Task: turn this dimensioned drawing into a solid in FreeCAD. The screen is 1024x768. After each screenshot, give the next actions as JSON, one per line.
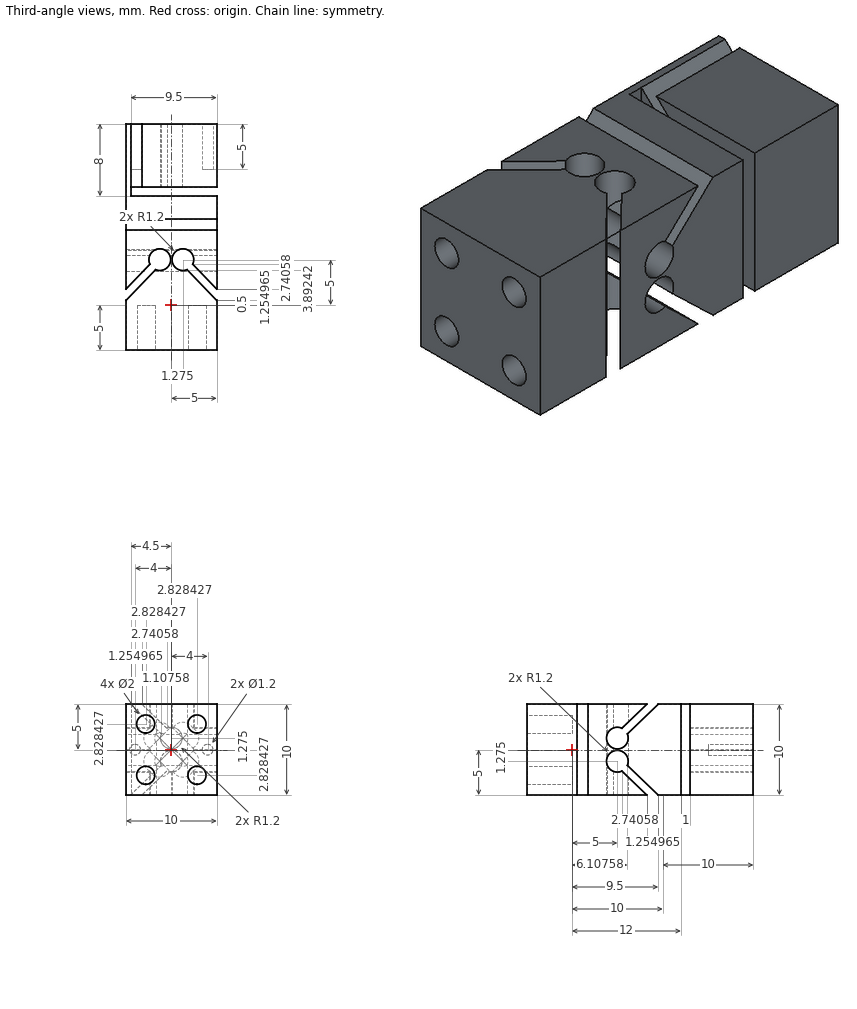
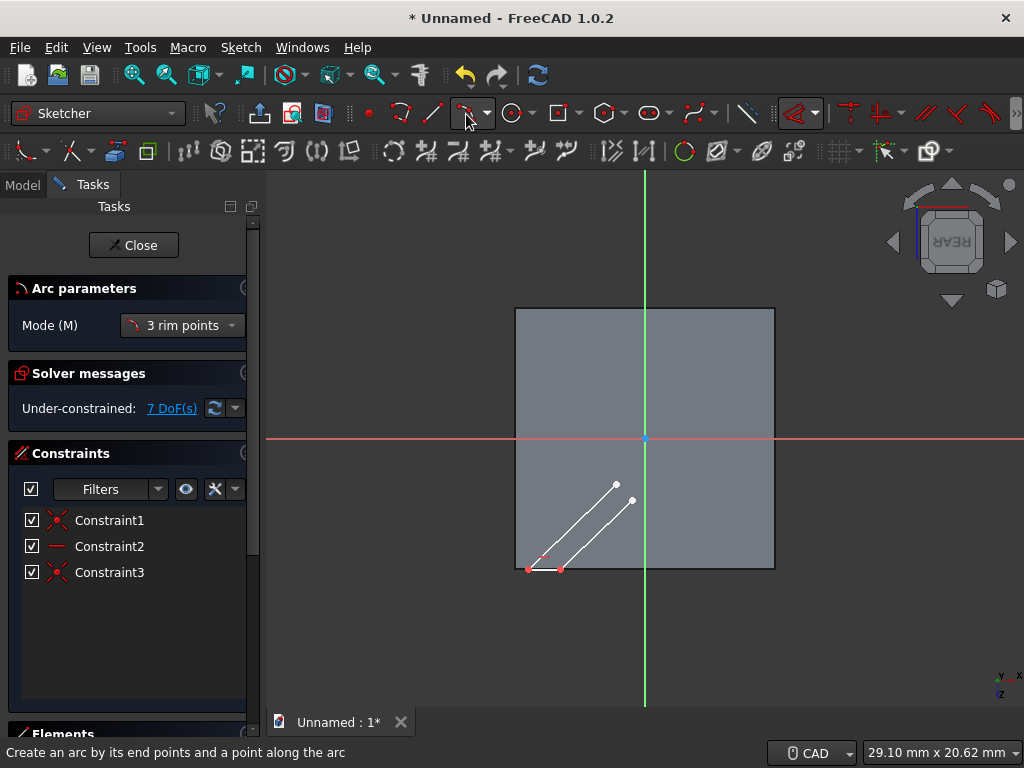
{"action": "left_click", "coordinate": [632, 501]}
{"action": "left_click", "coordinate": [616, 485]}
{"action": "left_click", "coordinate": [676, 465]}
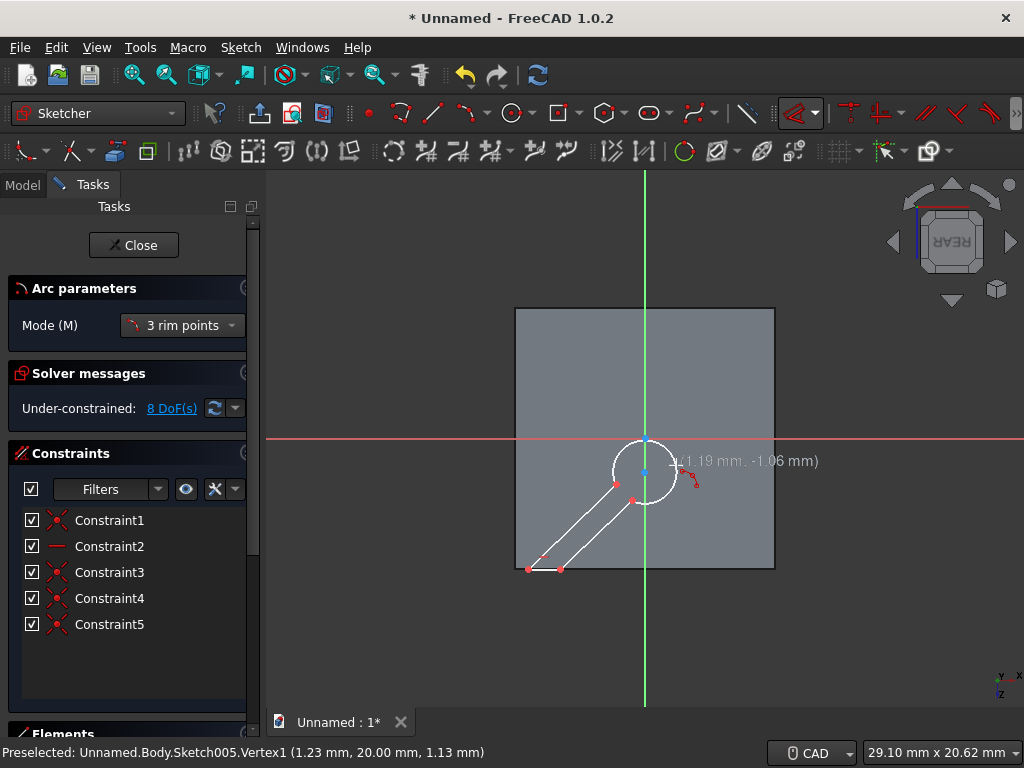
{"action": "left_click", "coordinate": [402, 114]}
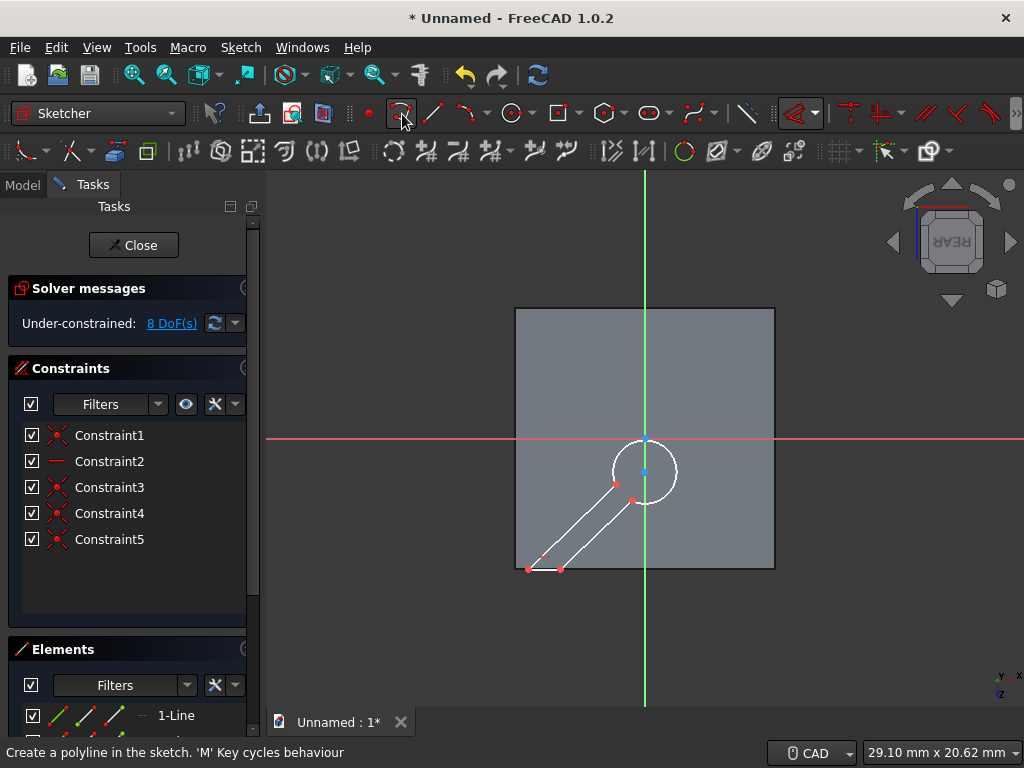
{"action": "left_click", "coordinate": [632, 377]}
{"action": "left_click", "coordinate": [560, 308]}
{"action": "left_click", "coordinate": [528, 308]}
{"action": "left_click", "coordinate": [616, 393]}
{"action": "right_click", "coordinate": [616, 393]}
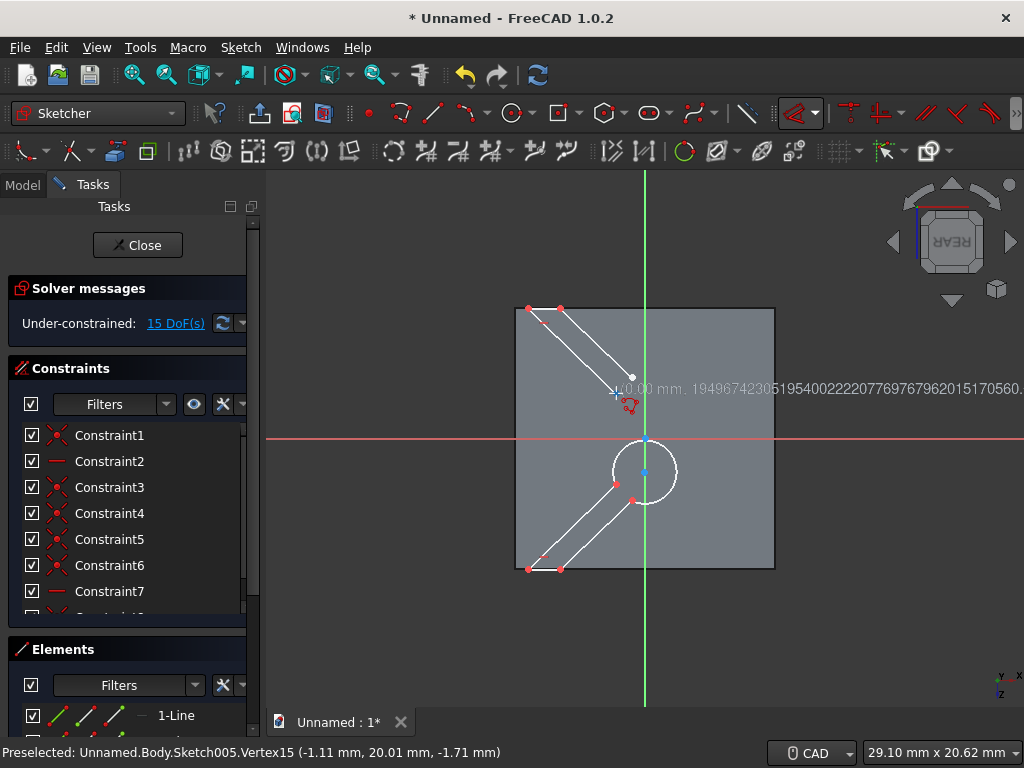
{"action": "left_click", "coordinate": [466, 114]}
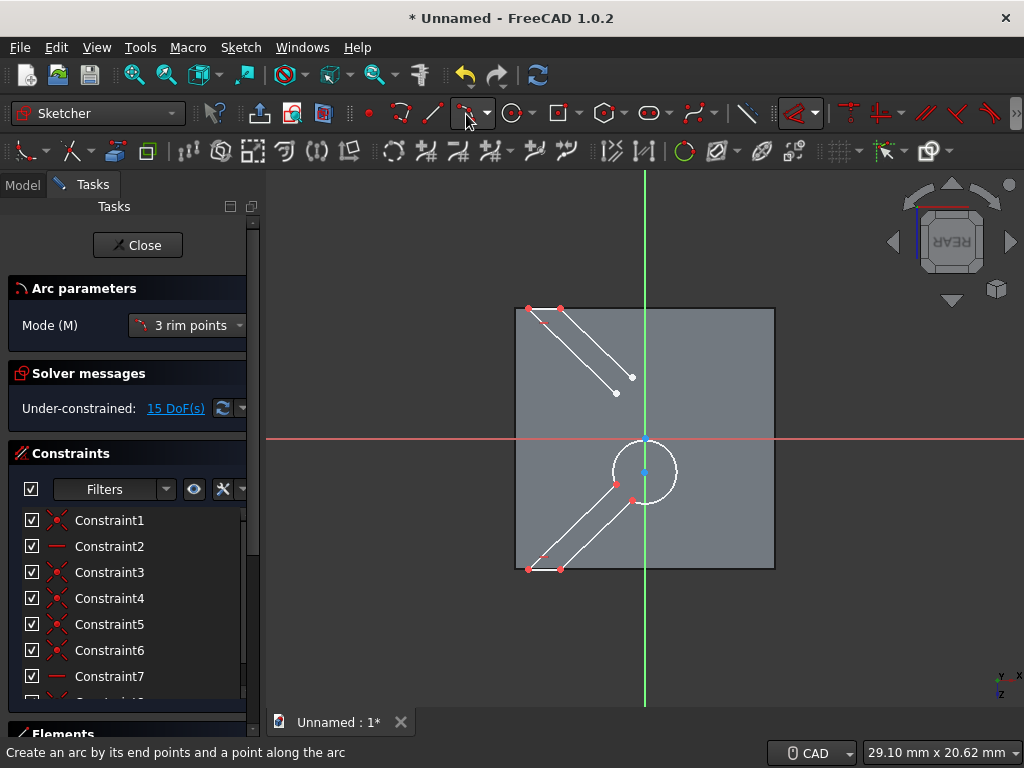
{"action": "left_click", "coordinate": [616, 394]}
{"action": "left_click", "coordinate": [632, 378]}
{"action": "left_click", "coordinate": [676, 412]}
{"action": "key", "text": "Escape"}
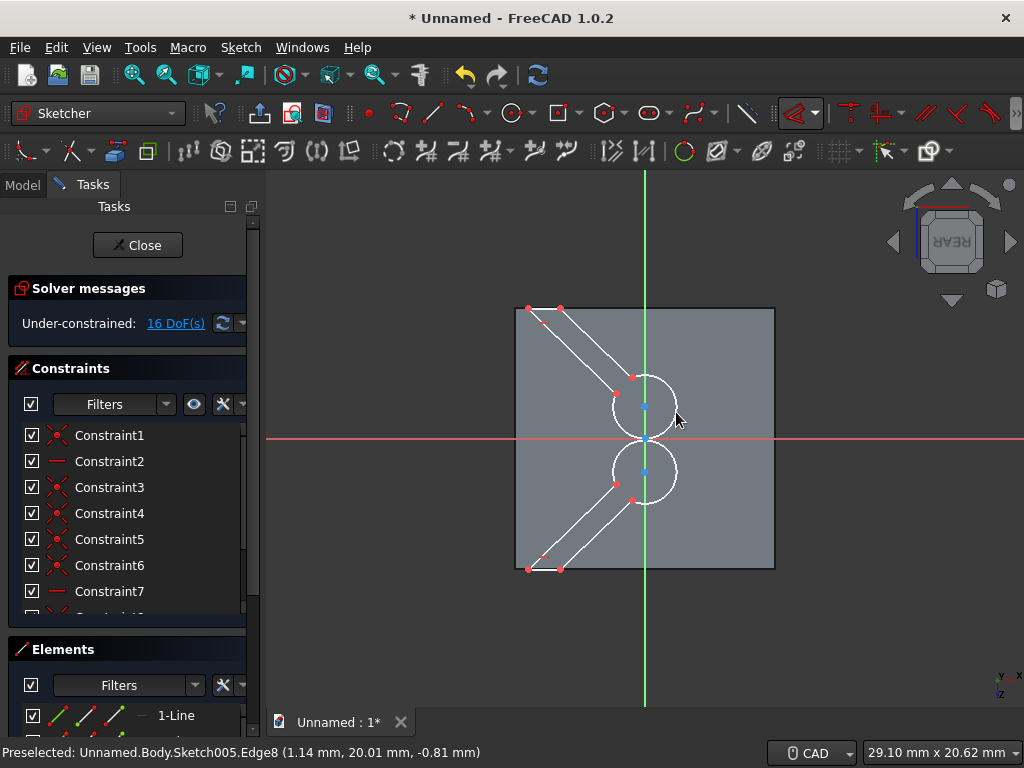
{"action": "left_click", "coordinate": [675, 482]}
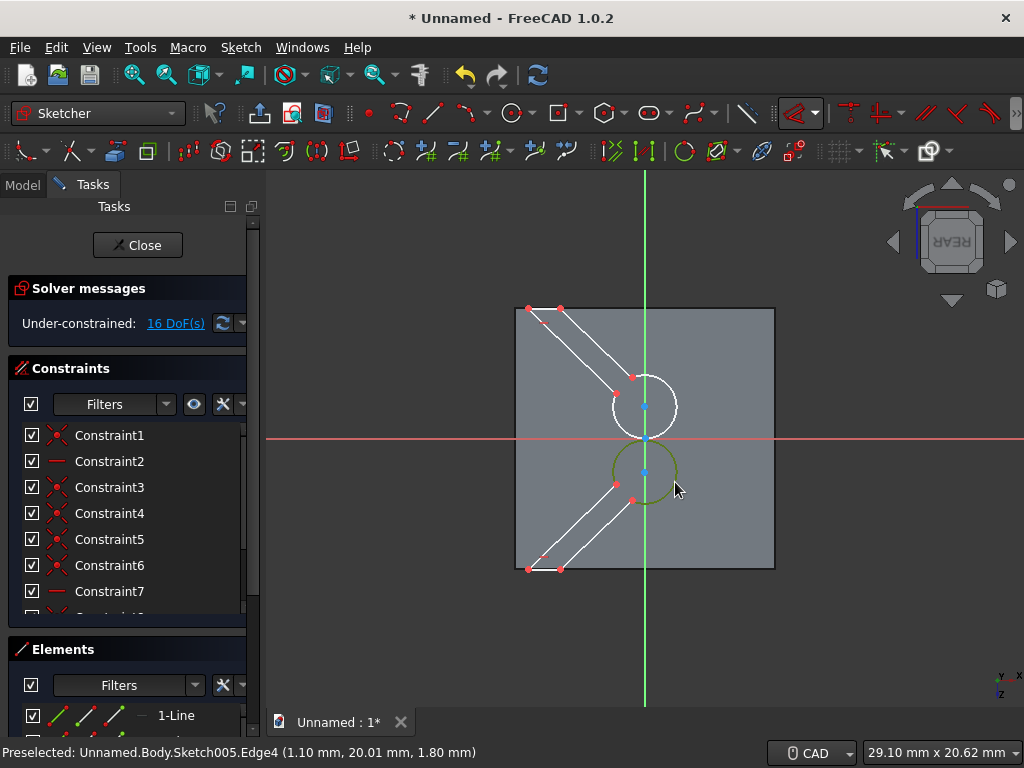
{"action": "left_click", "coordinate": [675, 397]}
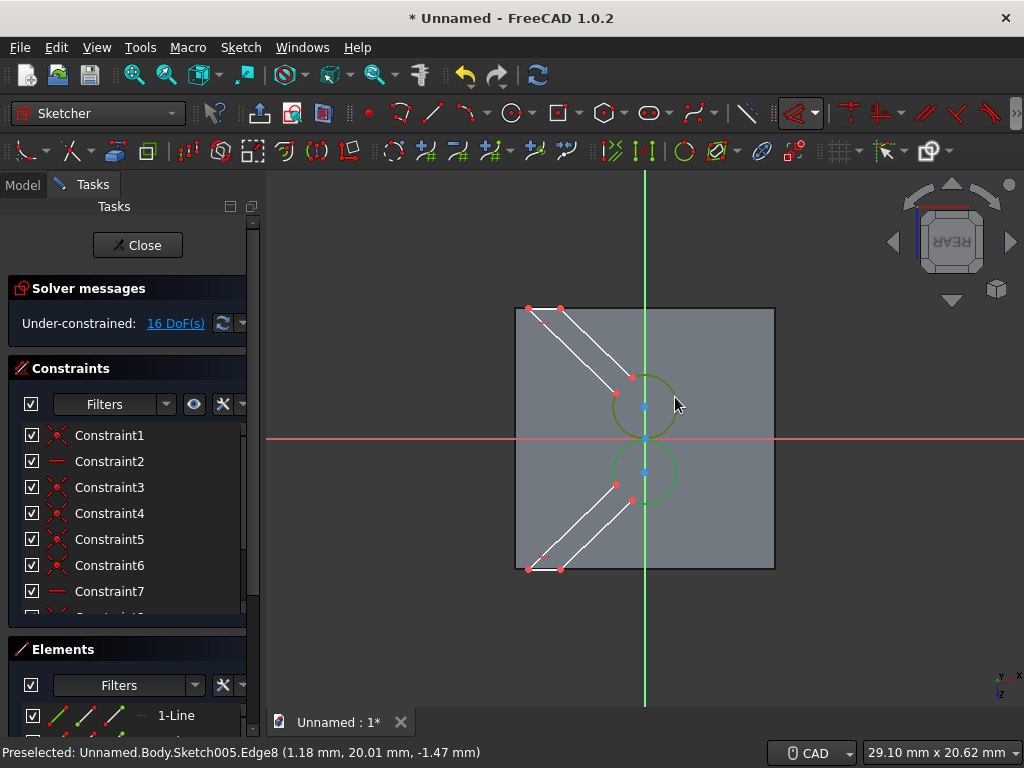
{"action": "key", "text": "e"}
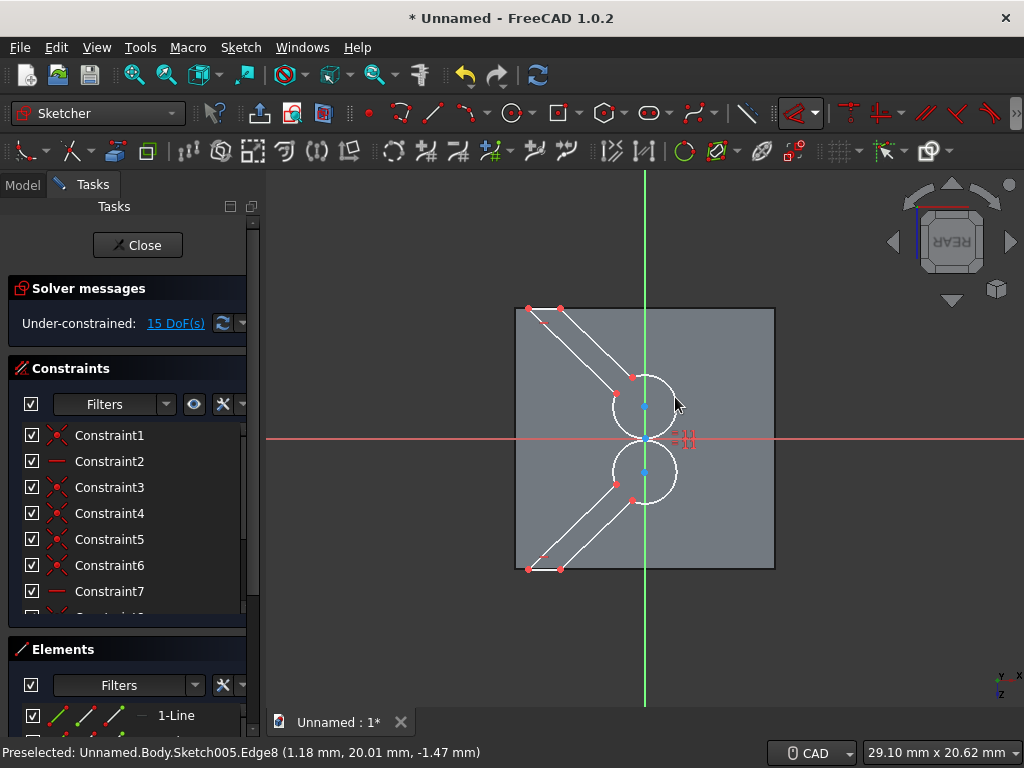
{"action": "left_click", "coordinate": [645, 472]}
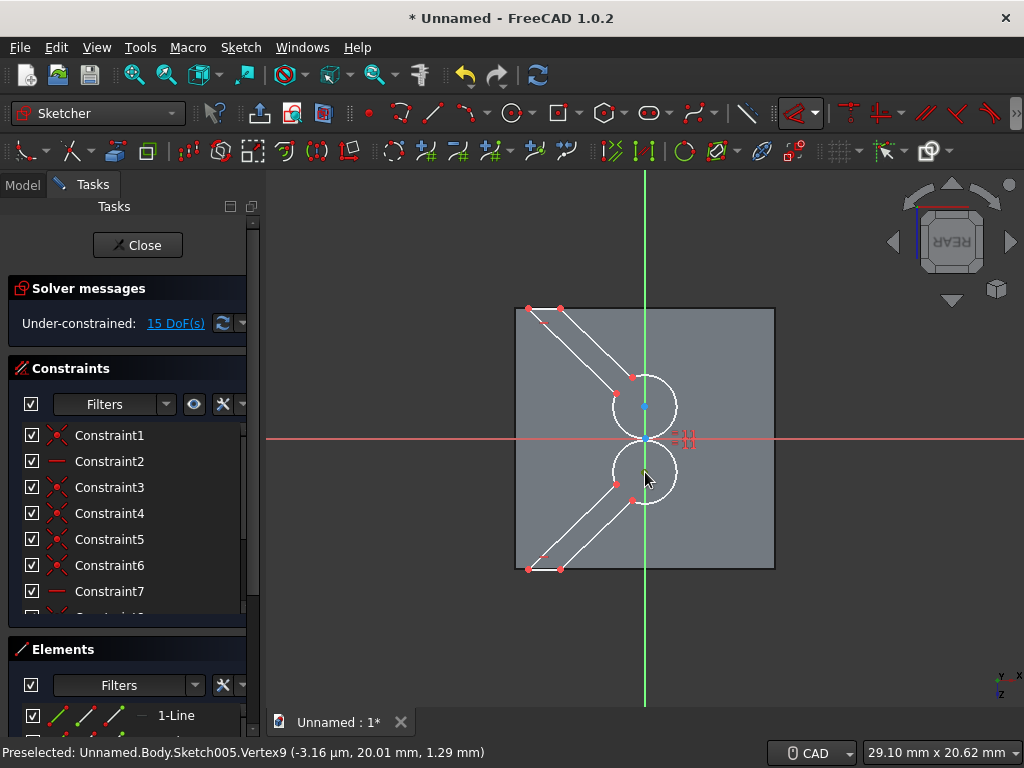
{"action": "left_click", "coordinate": [645, 645]}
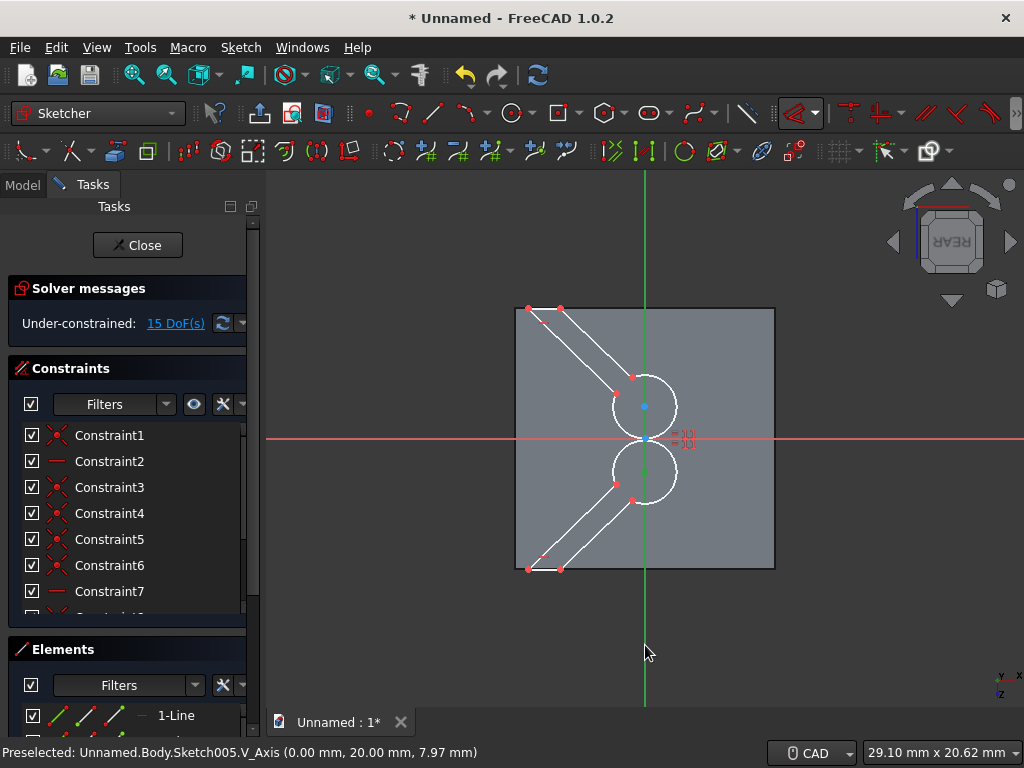
{"action": "left_click", "coordinate": [850, 114]}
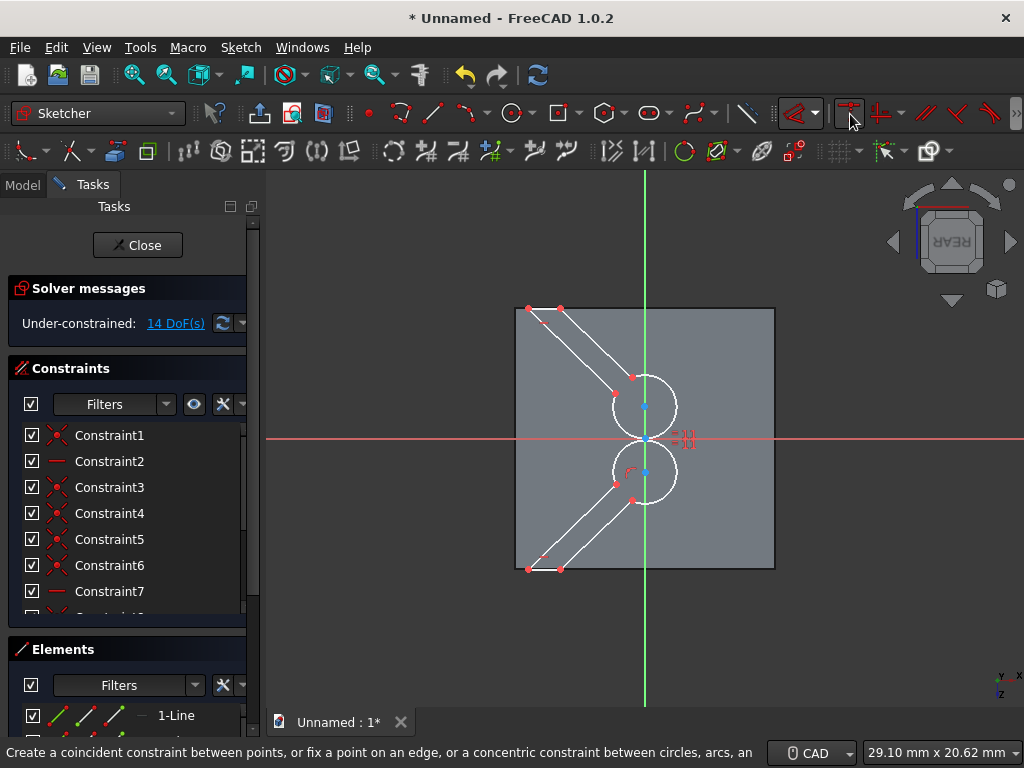
{"action": "left_click", "coordinate": [645, 407]}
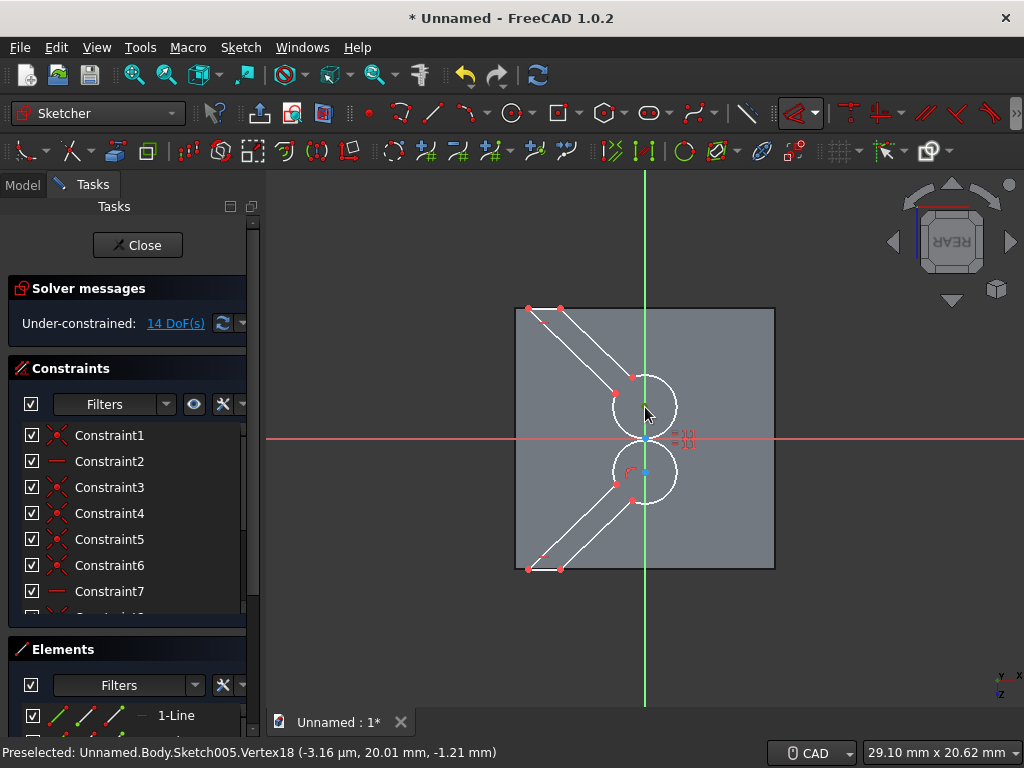
{"action": "left_click", "coordinate": [645, 645]}